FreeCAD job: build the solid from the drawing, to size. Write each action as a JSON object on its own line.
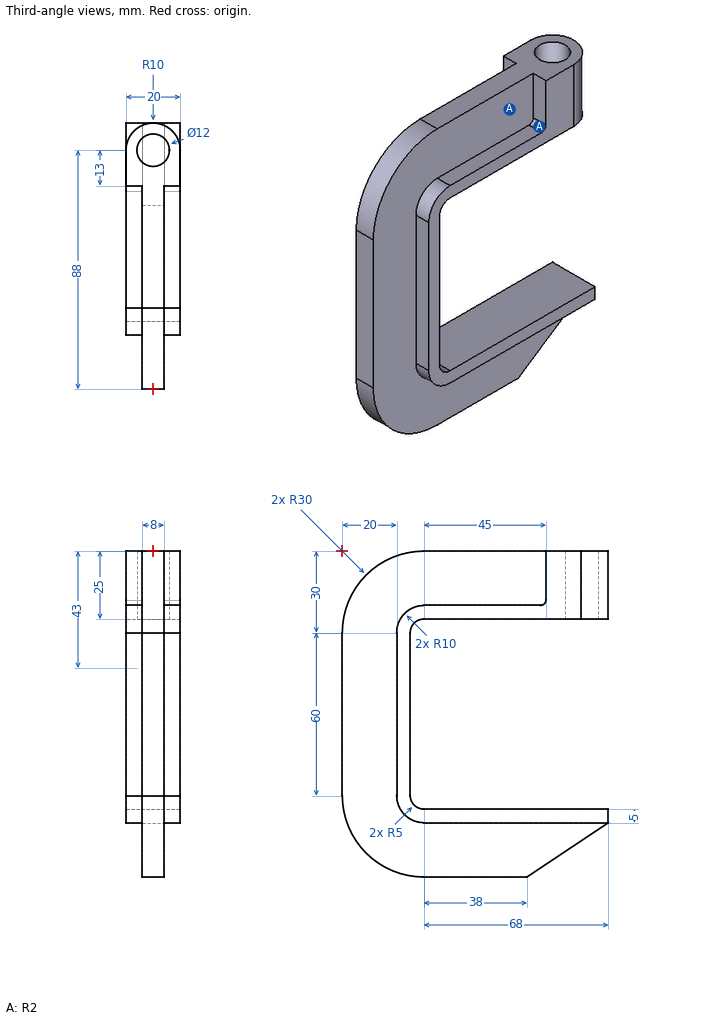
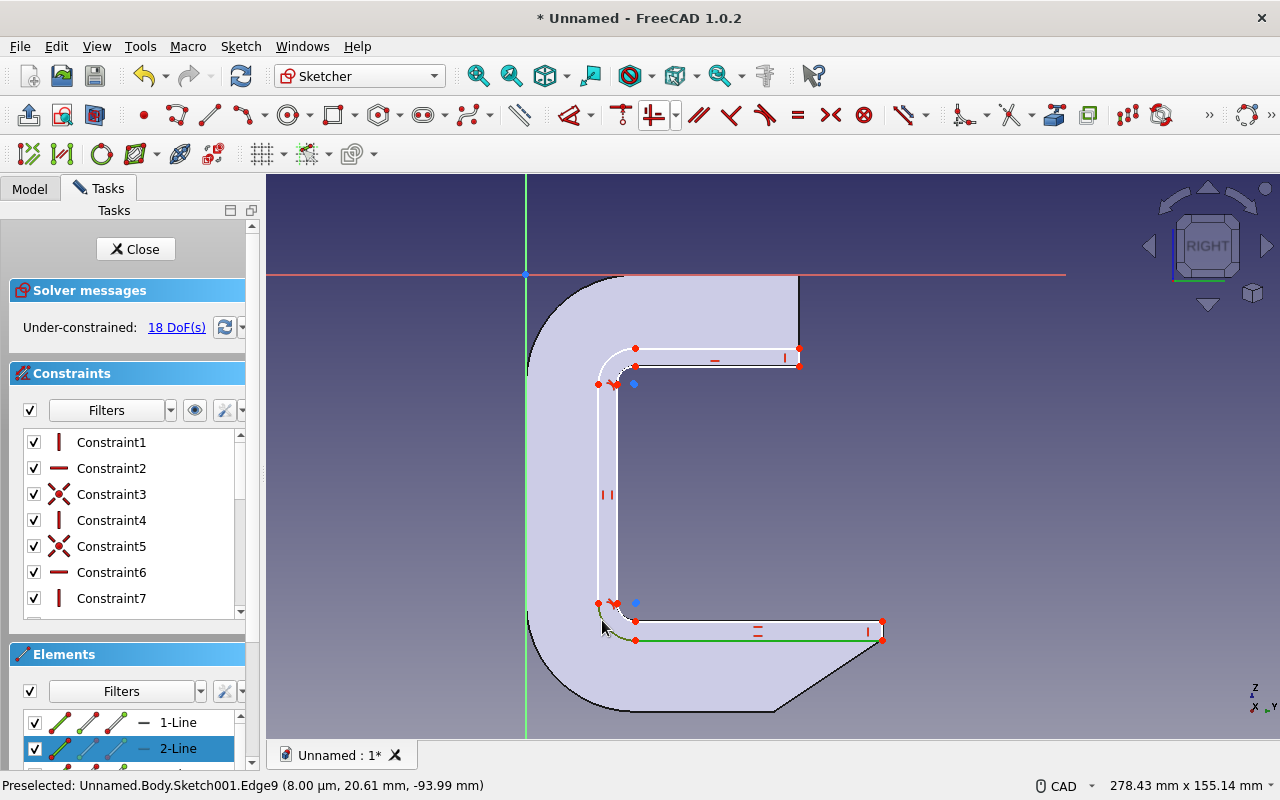
{"action": "key", "text": "t"}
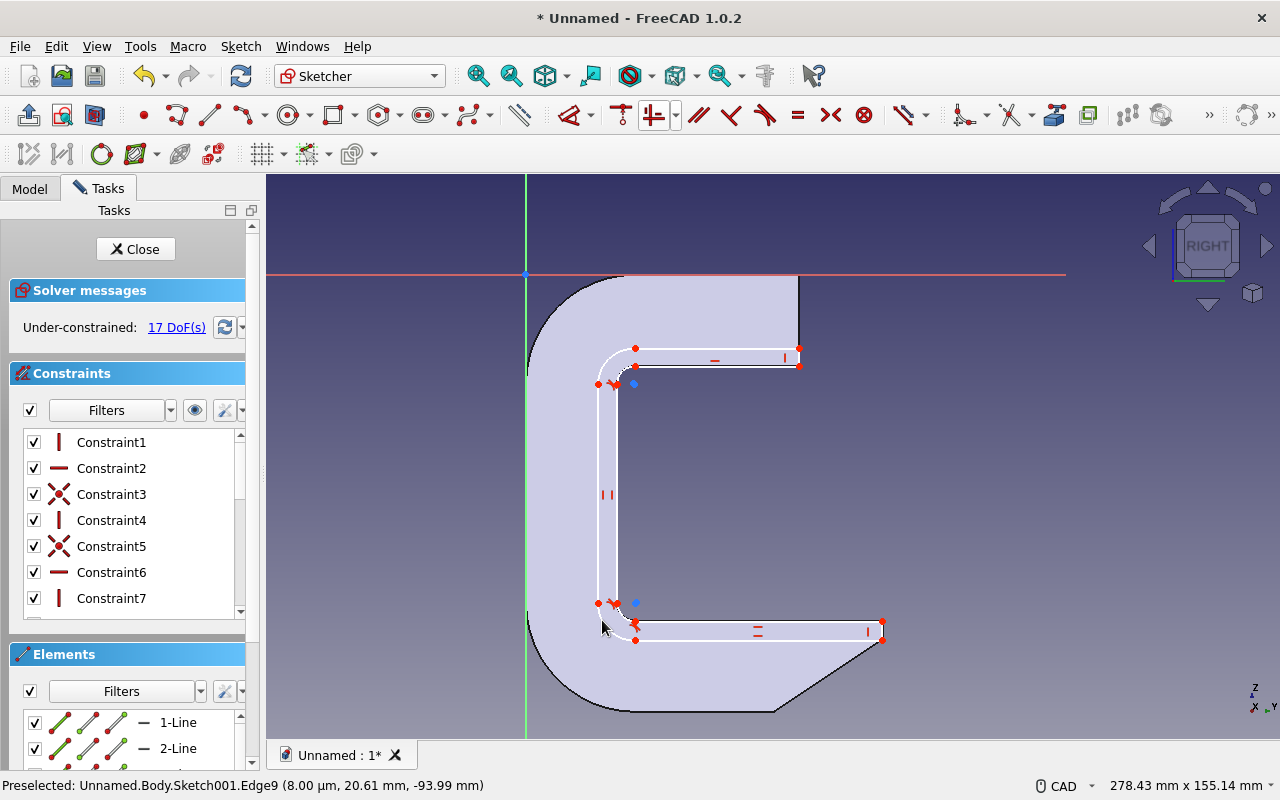
{"action": "left_click", "coordinate": [808, 622]}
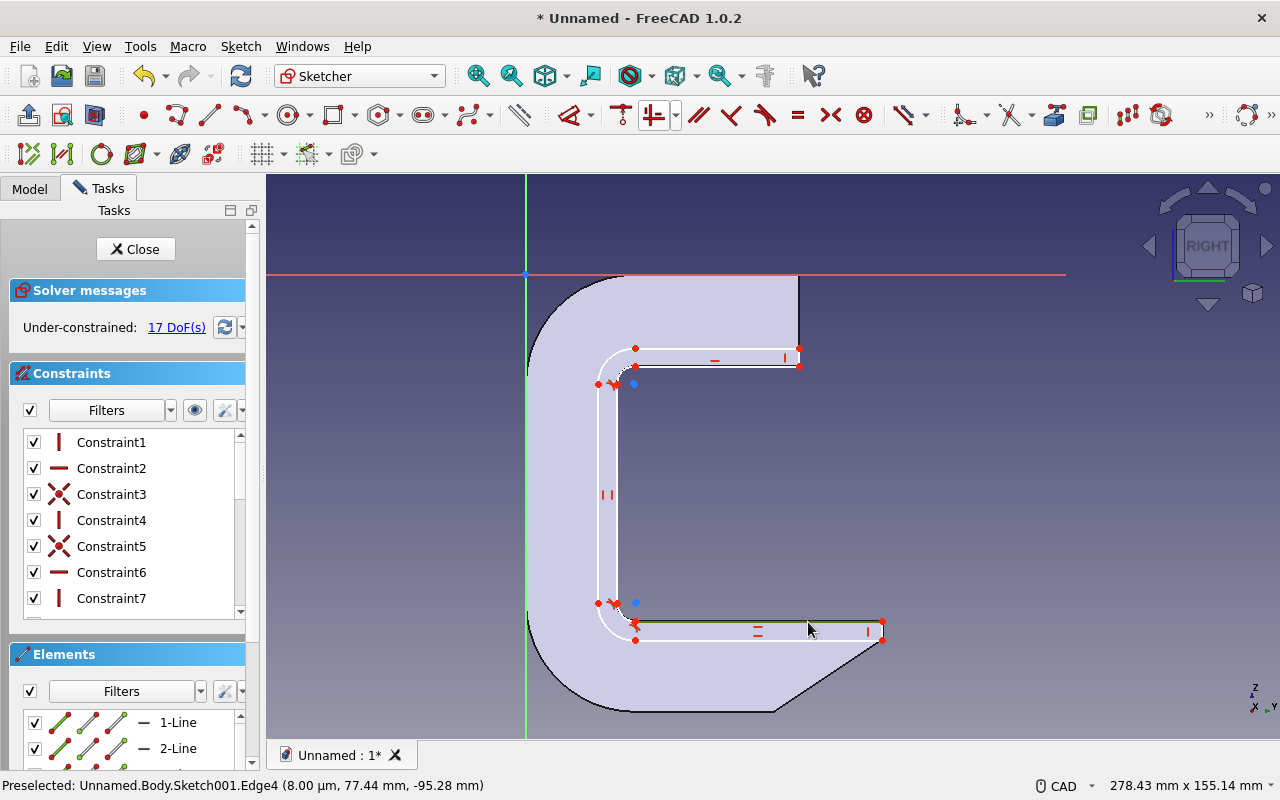
{"action": "left_click", "coordinate": [623, 616]}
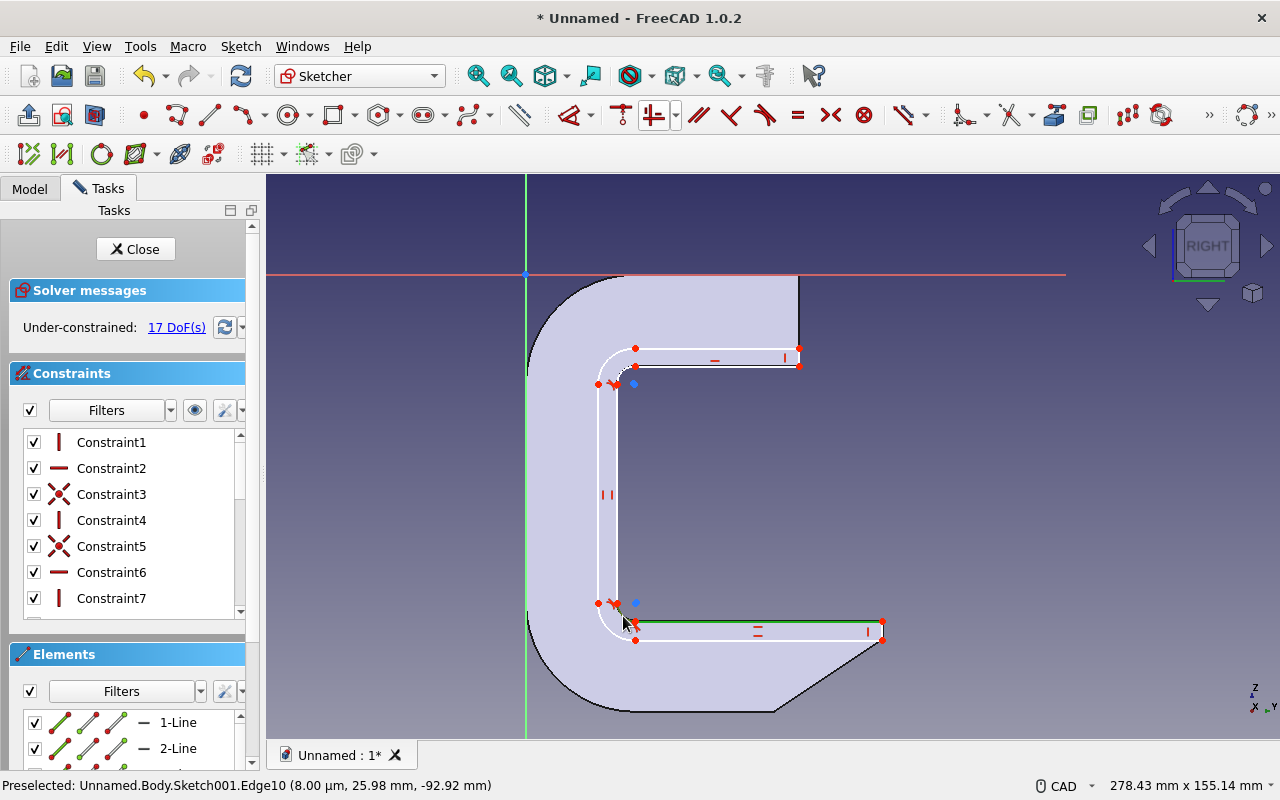
{"action": "key", "text": "t"}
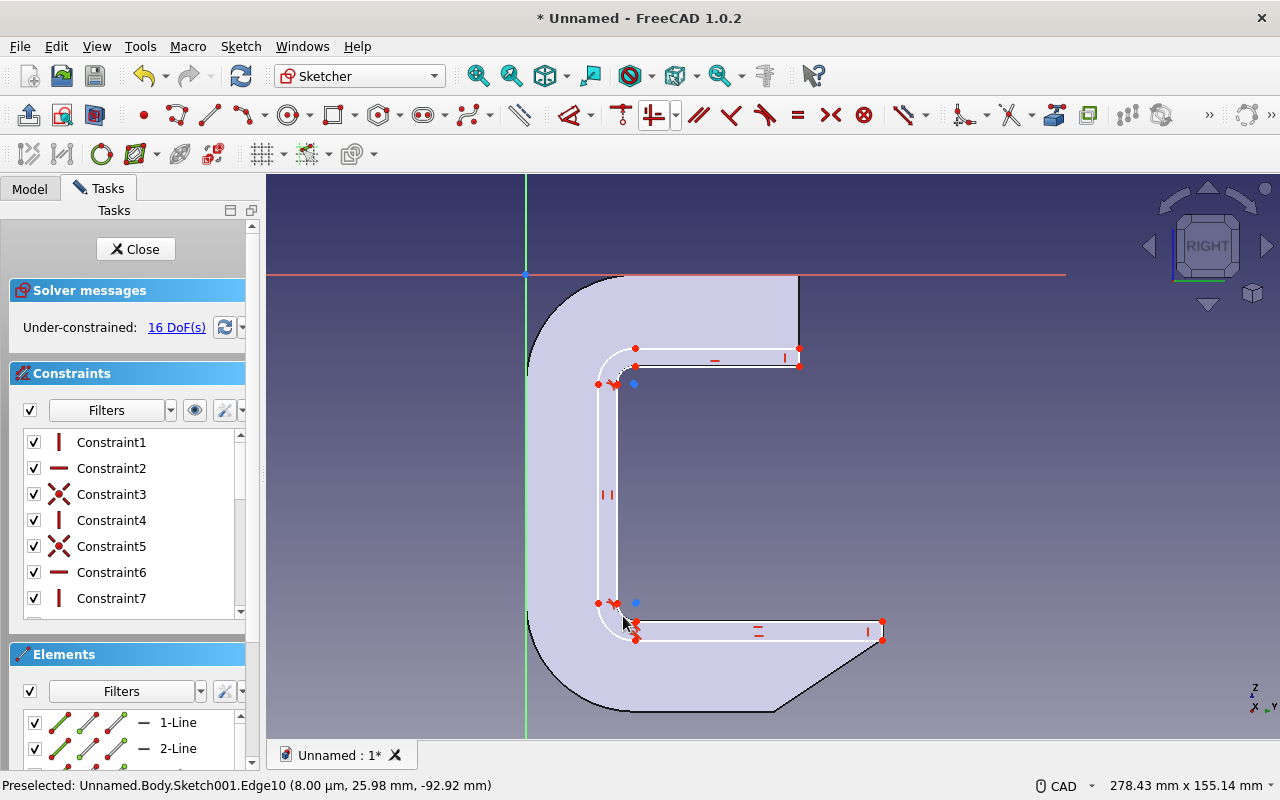
{"action": "left_click", "coordinate": [617, 538]}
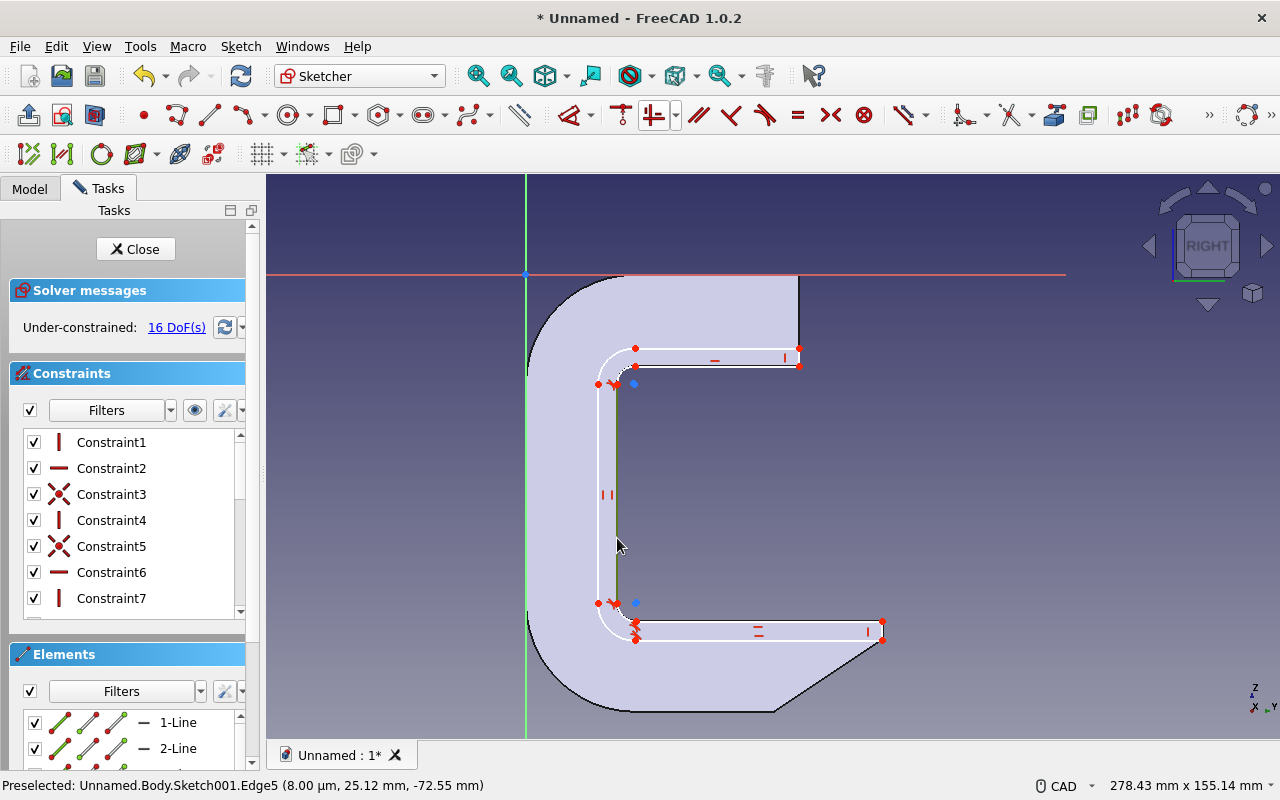
{"action": "left_click", "coordinate": [623, 617]}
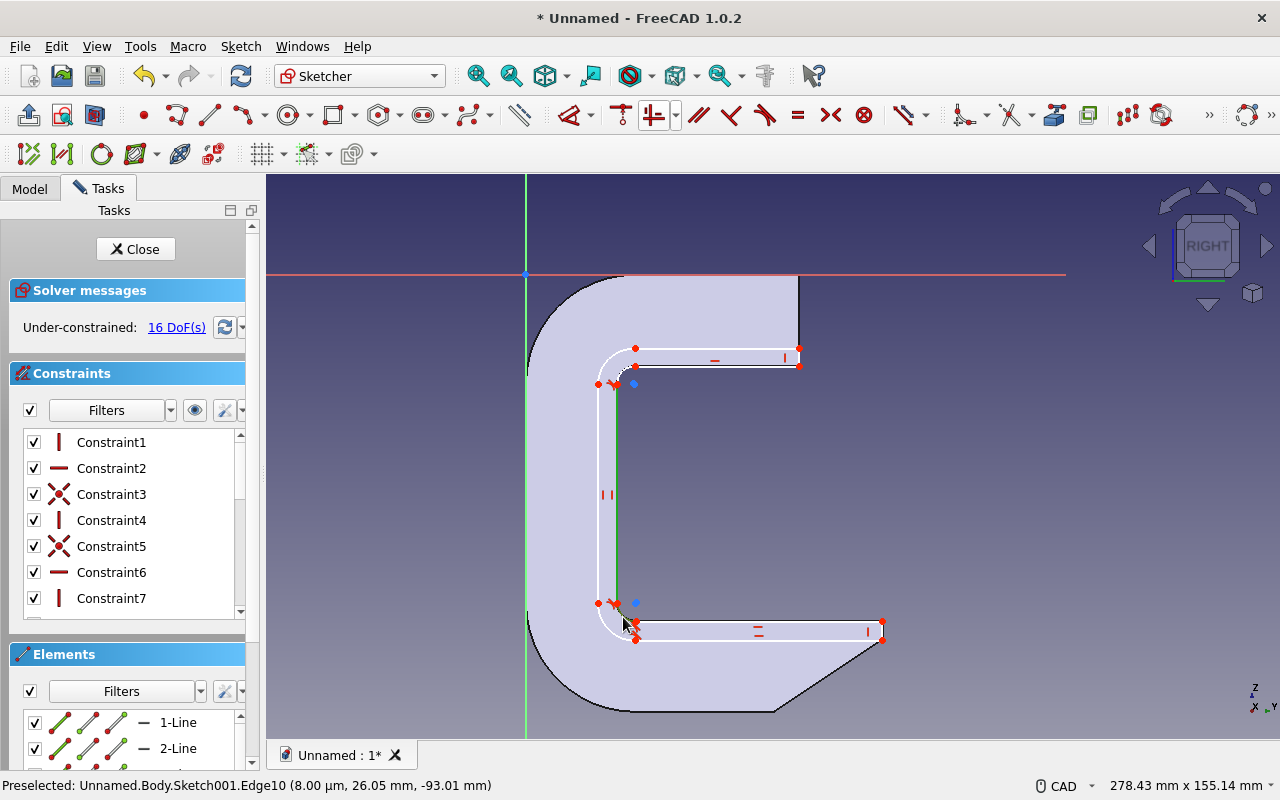
{"action": "key", "text": "t"}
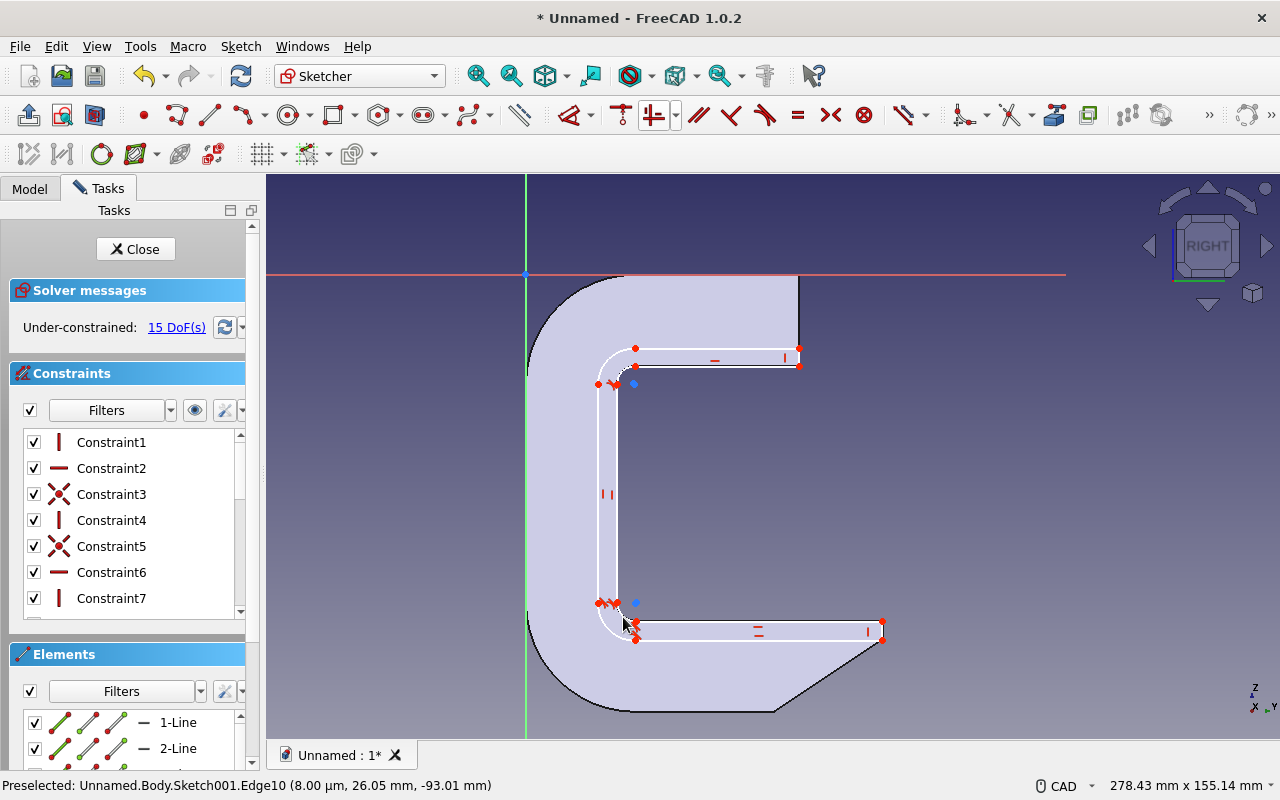
{"action": "left_click", "coordinate": [617, 537]}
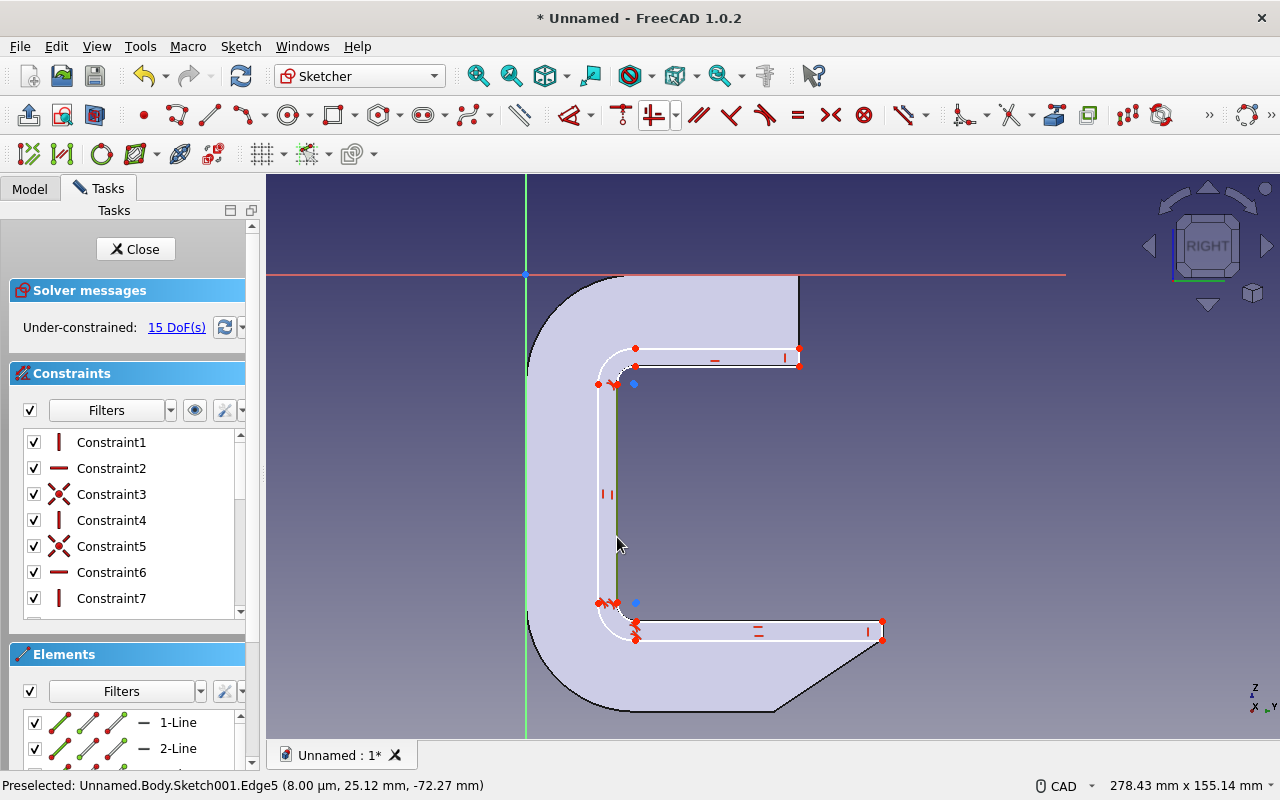
{"action": "left_click", "coordinate": [622, 372]}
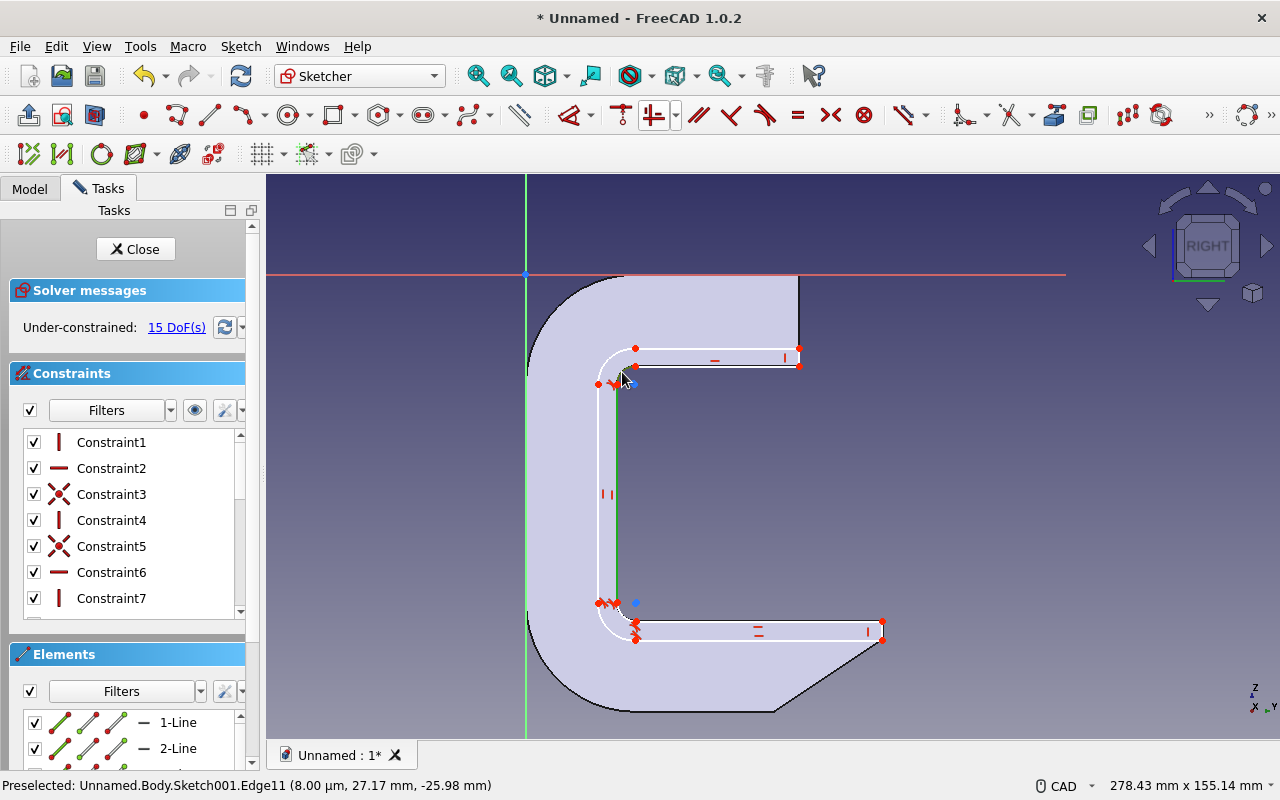
{"action": "key", "text": "t"}